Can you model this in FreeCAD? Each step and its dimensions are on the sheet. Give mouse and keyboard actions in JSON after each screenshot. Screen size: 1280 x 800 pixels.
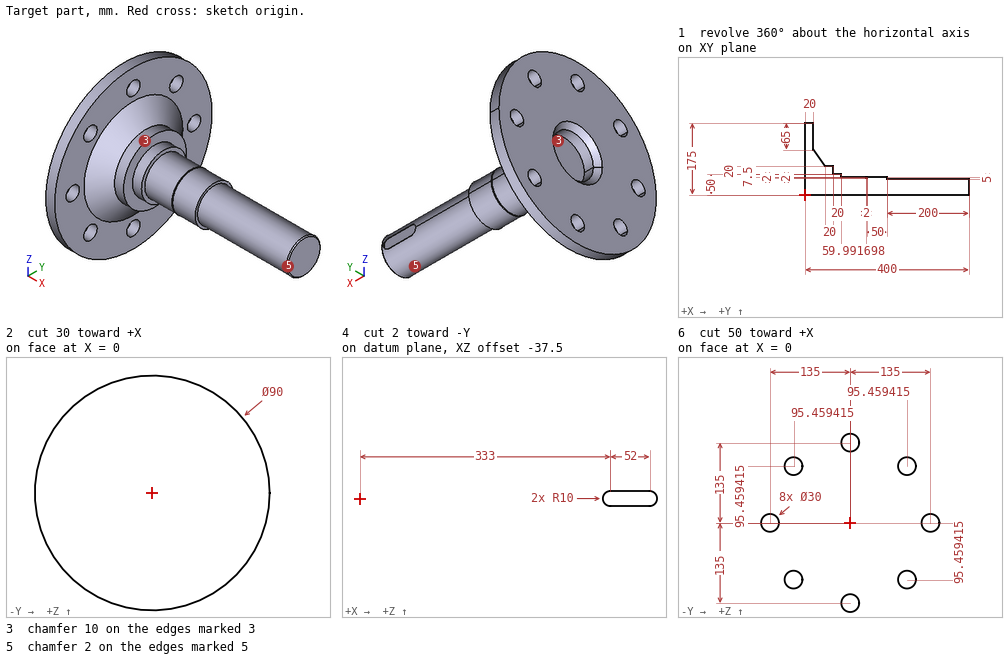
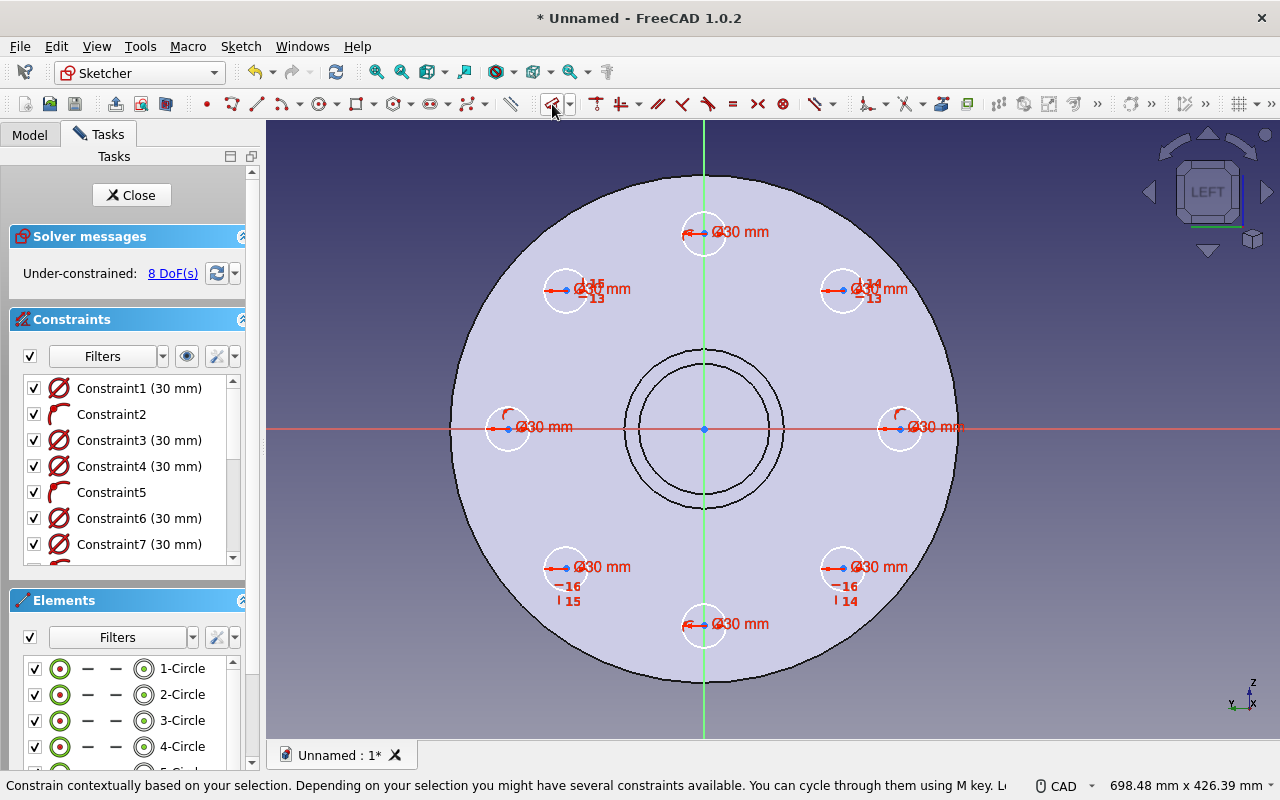
{"action": "left_click", "coordinate": [508, 429]}
{"action": "left_click", "coordinate": [606, 463]}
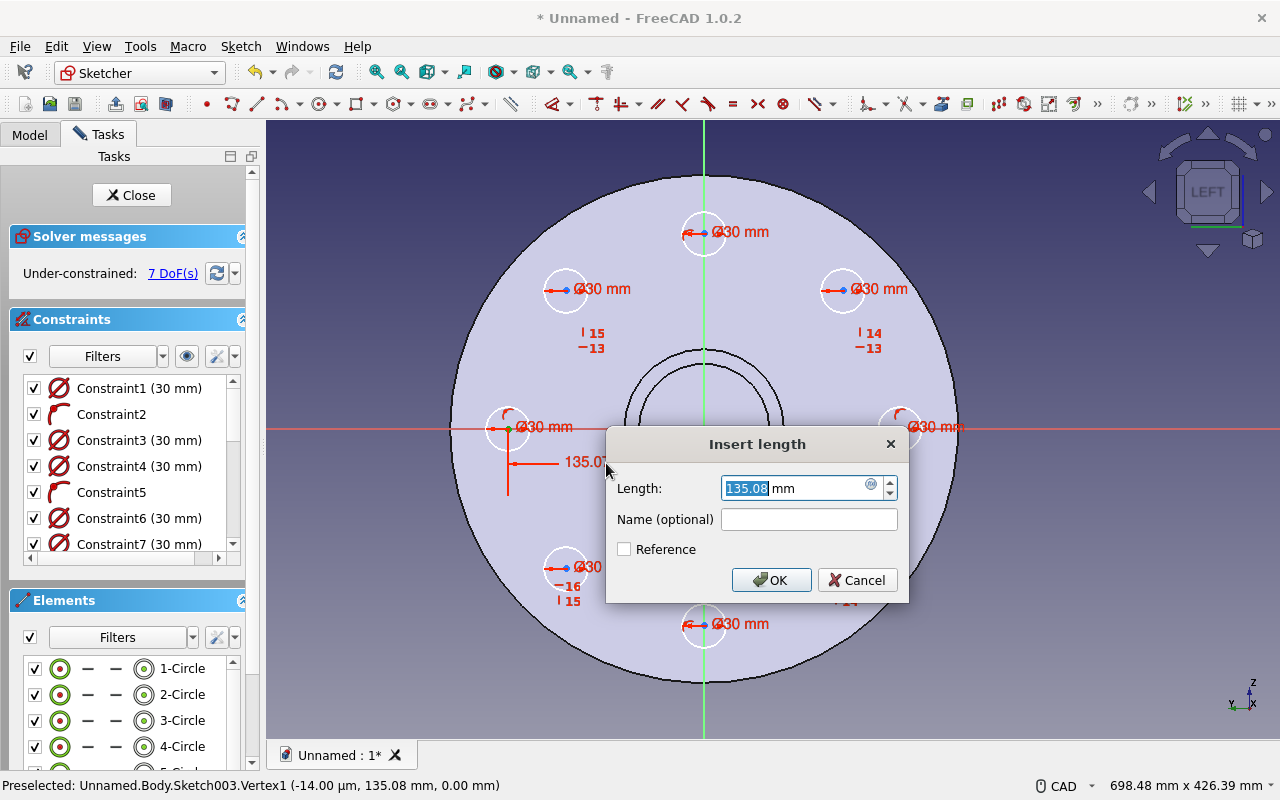
{"action": "type", "text": "135"}
{"action": "key", "text": "Return"}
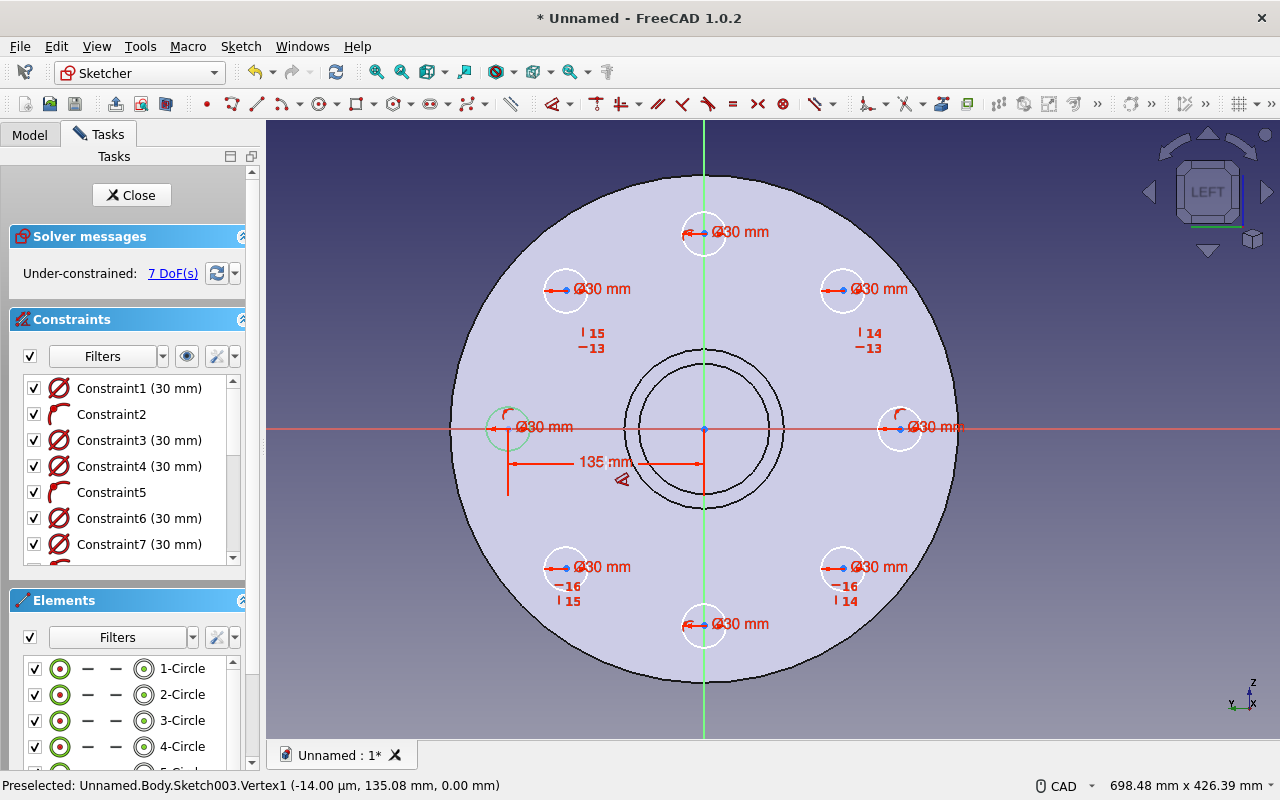
{"action": "left_click", "coordinate": [704, 234]}
{"action": "left_click", "coordinate": [738, 332]}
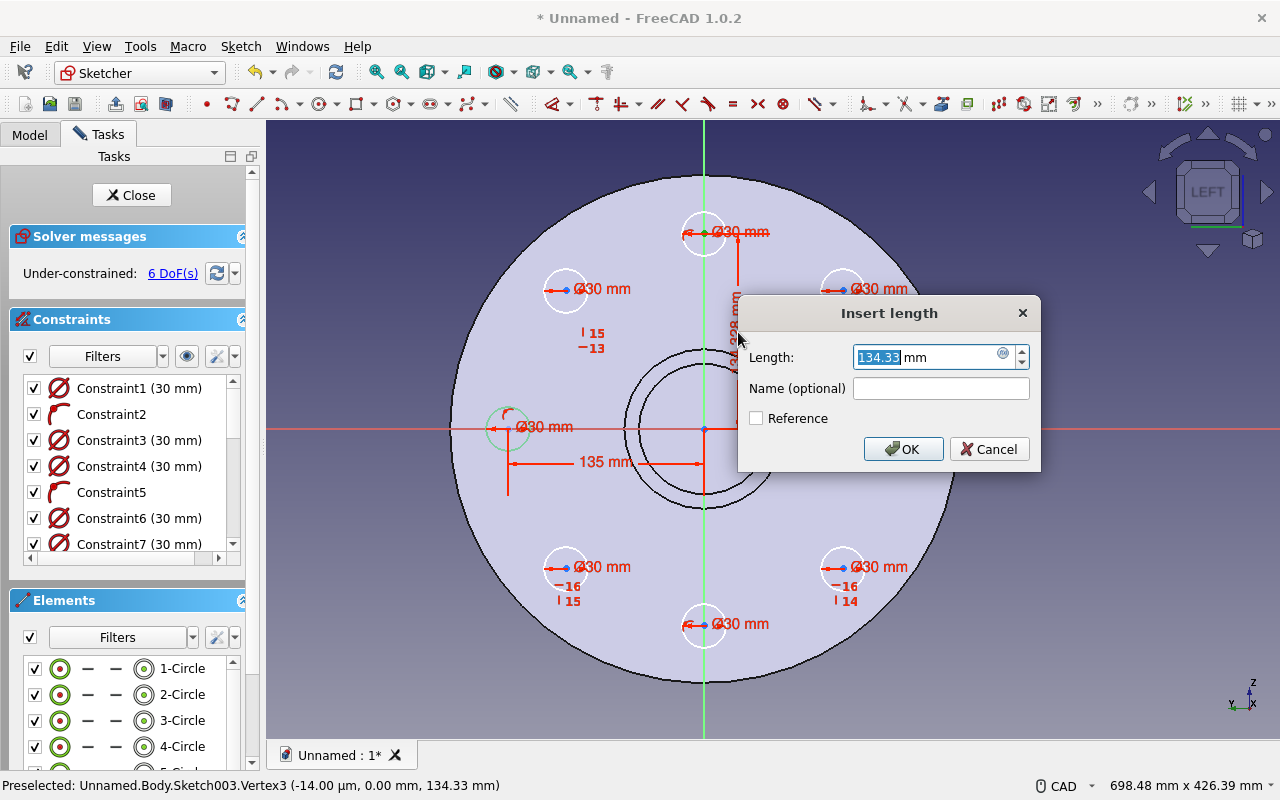
{"action": "type", "text": "135"}
{"action": "key", "text": "Return"}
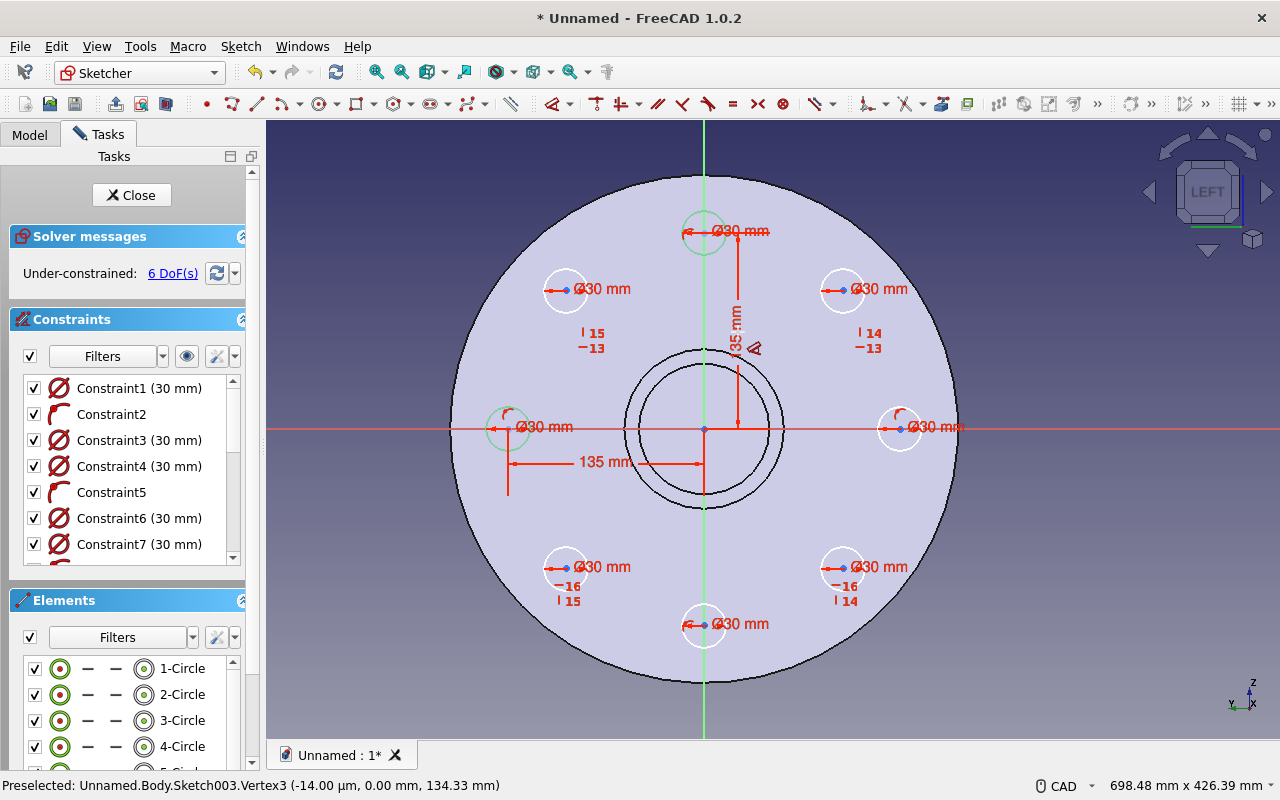
{"action": "left_click", "coordinate": [900, 429]}
{"action": "left_click", "coordinate": [802, 463]}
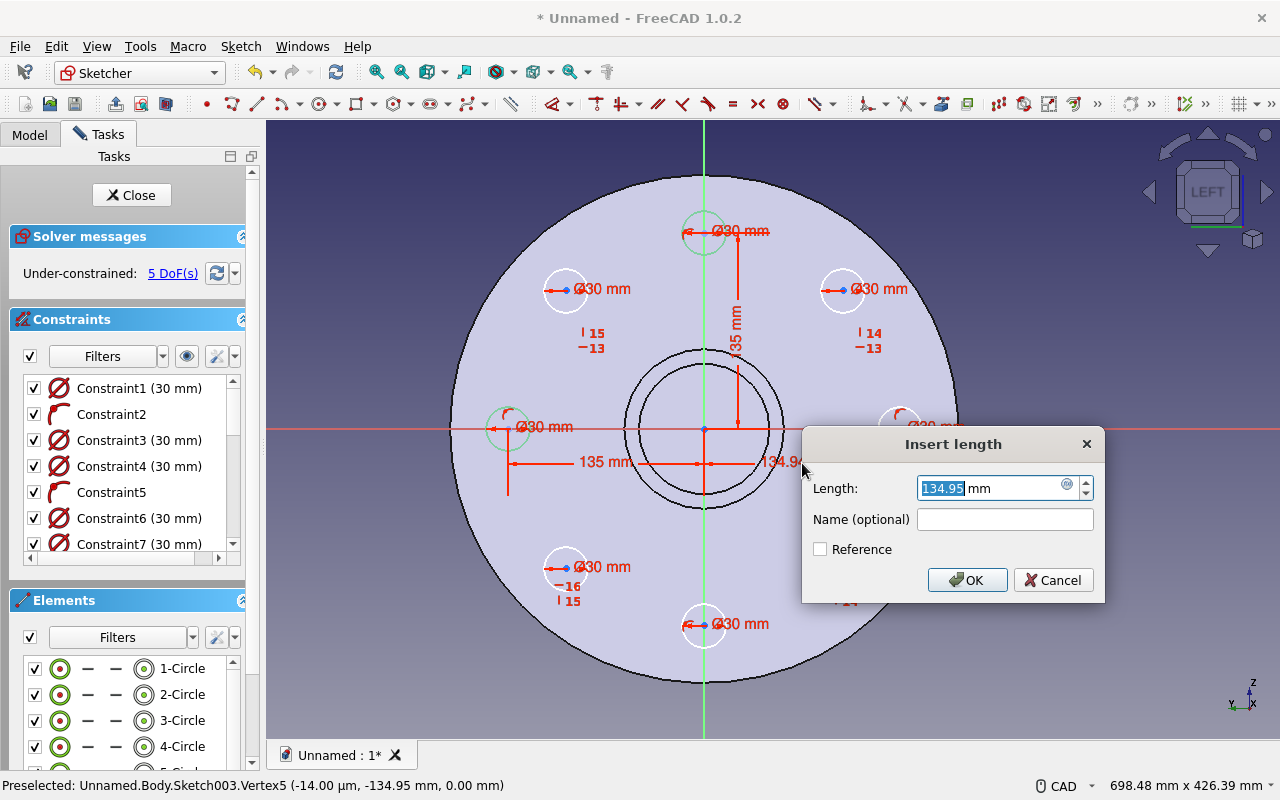
{"action": "type", "text": "135"}
{"action": "key", "text": "Return"}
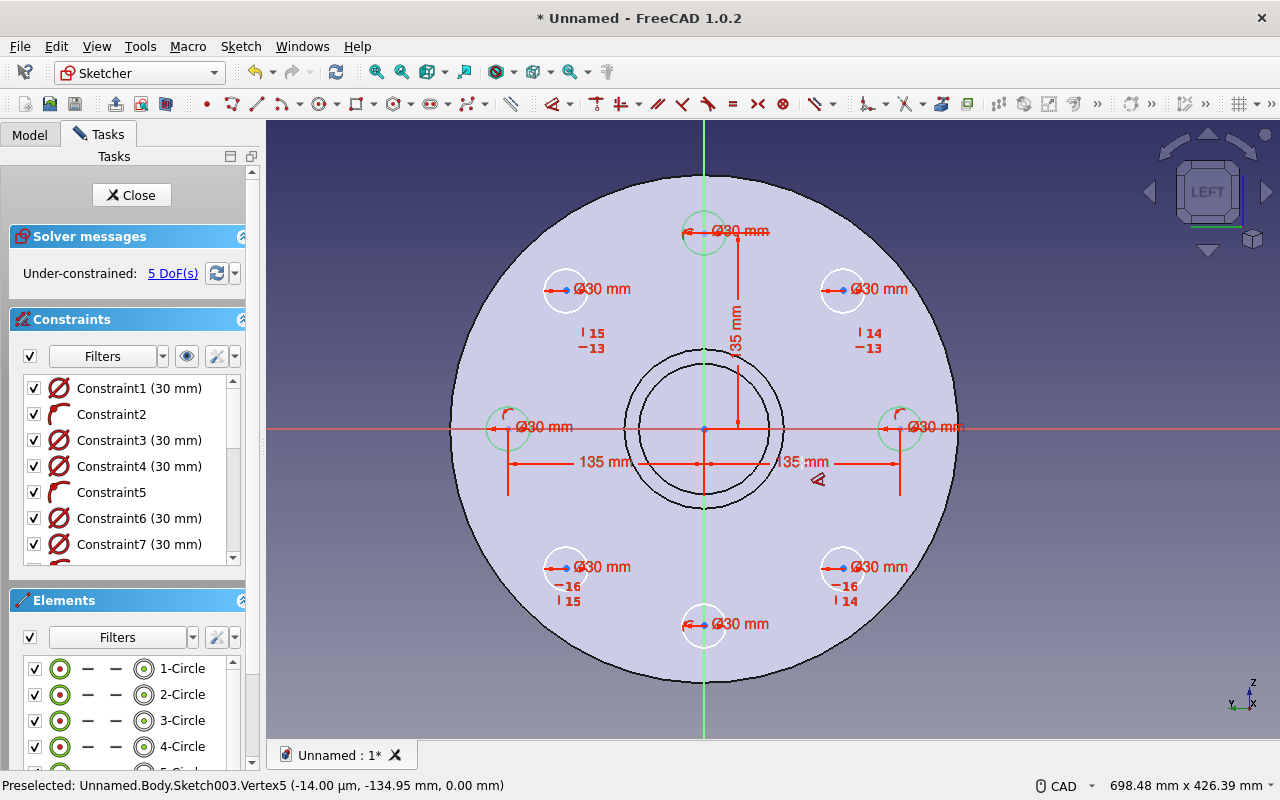
{"action": "left_click", "coordinate": [704, 626]}
{"action": "left_click", "coordinate": [738, 528]}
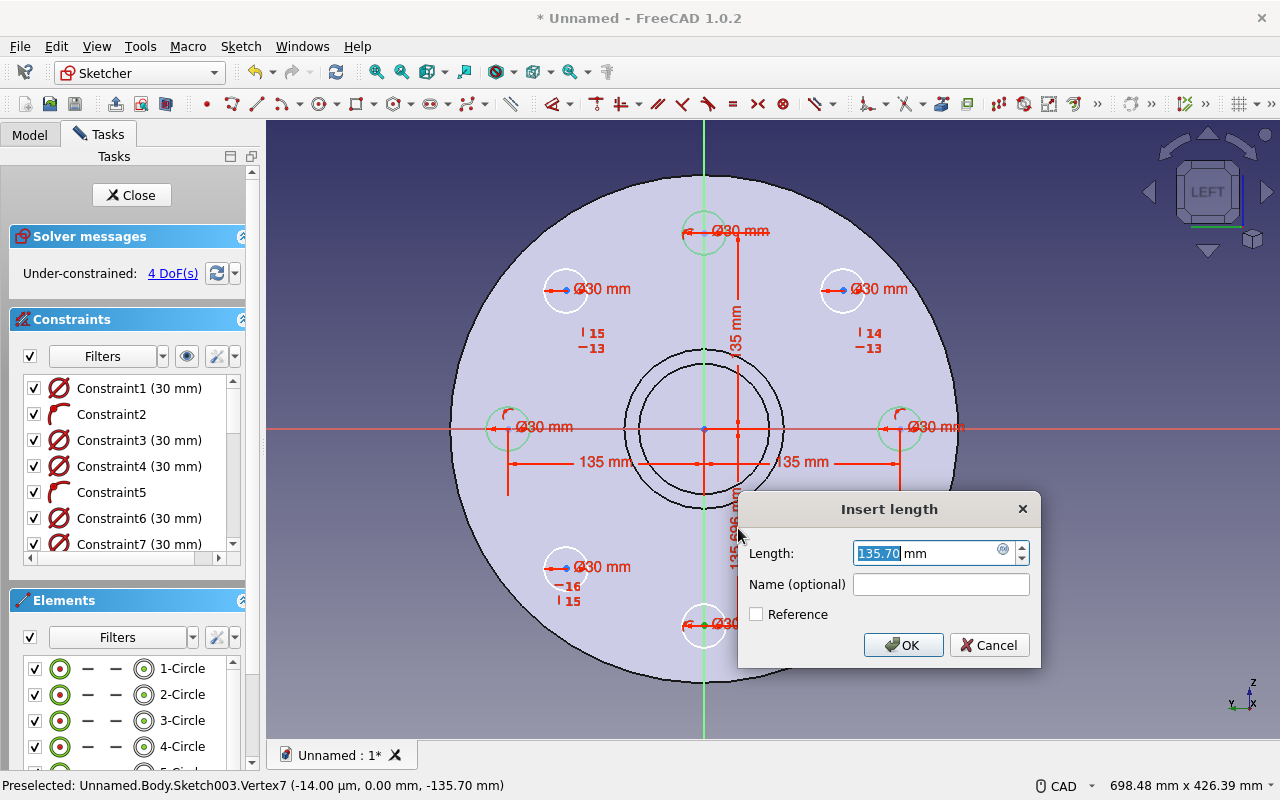
{"action": "type", "text": "135"}
{"action": "key", "text": "Return"}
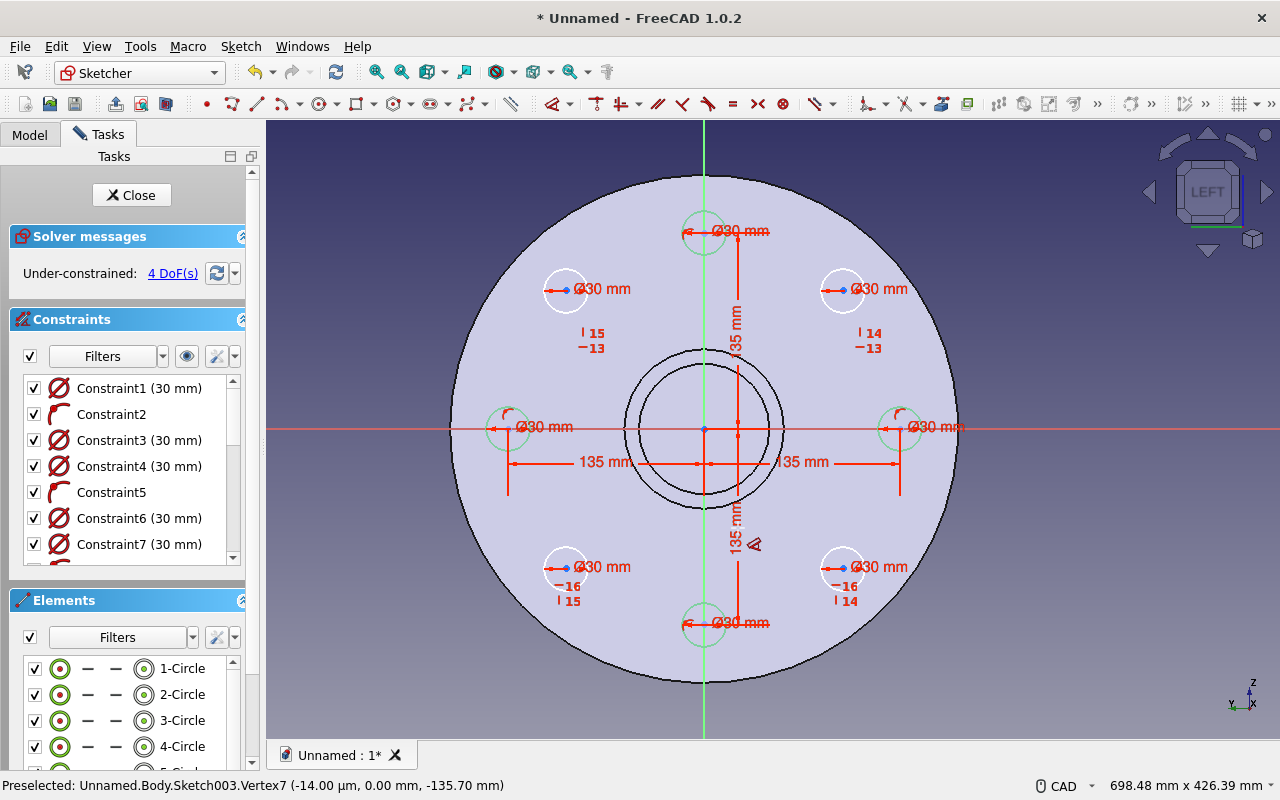
{"action": "left_click", "coordinate": [566, 291]}
{"action": "left_click", "coordinate": [635, 257]}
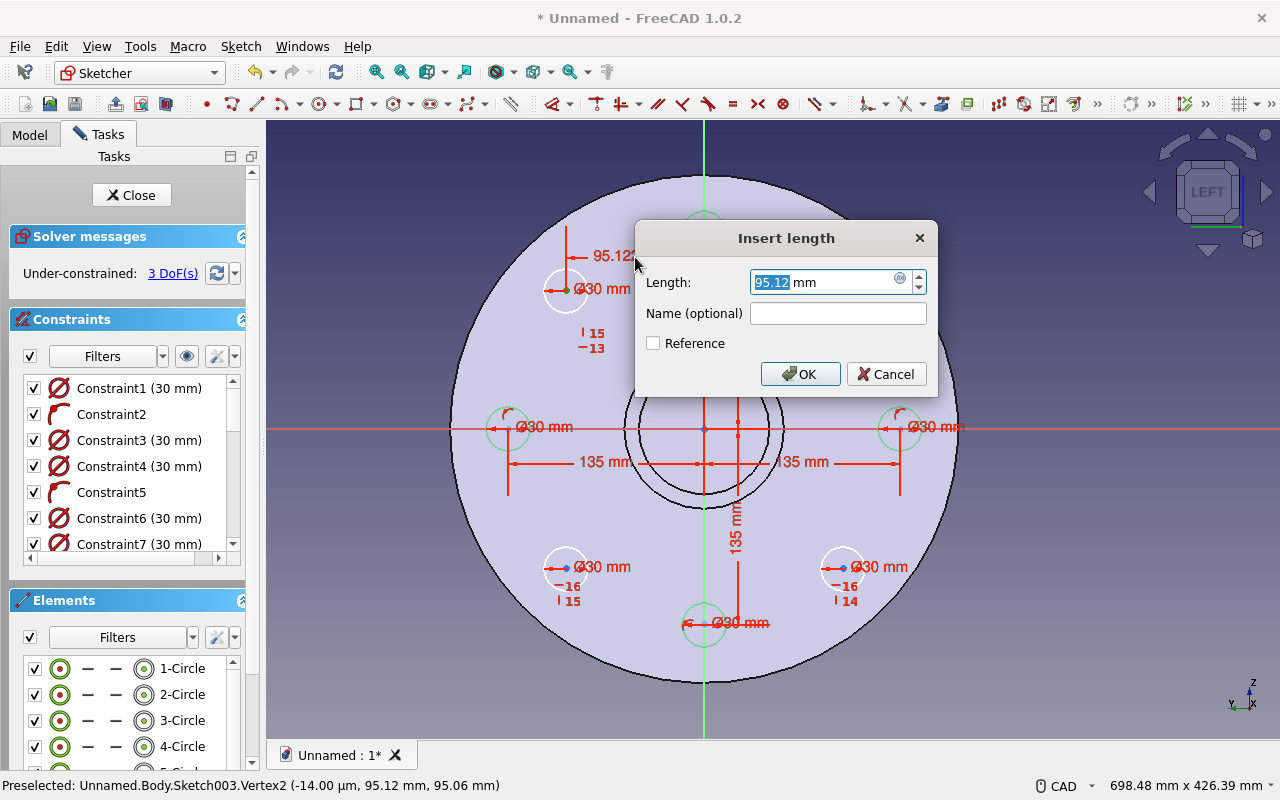
{"action": "type", "text": "95.459415"}
{"action": "key", "text": "Return"}